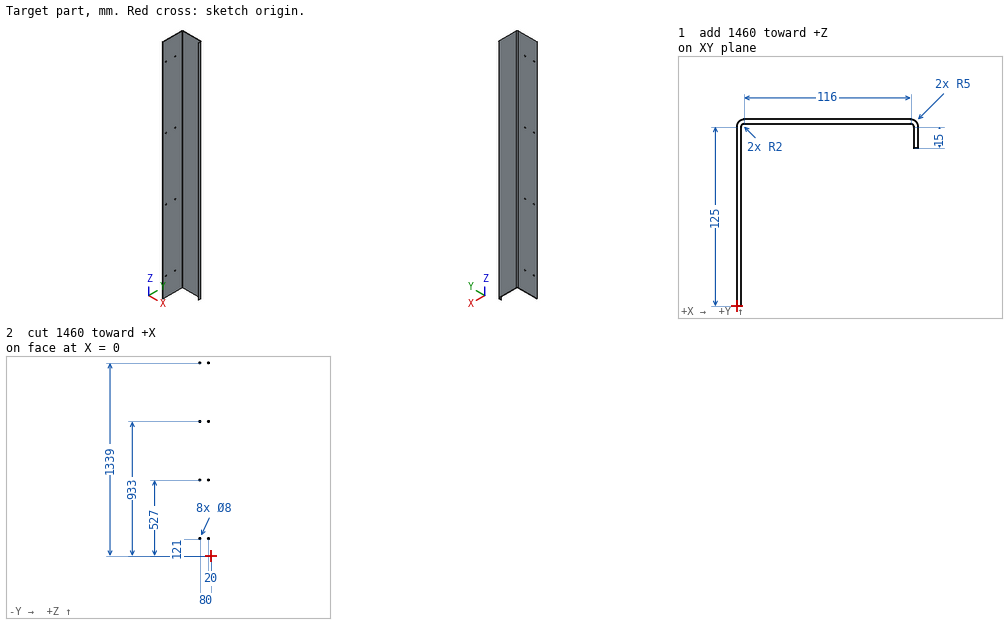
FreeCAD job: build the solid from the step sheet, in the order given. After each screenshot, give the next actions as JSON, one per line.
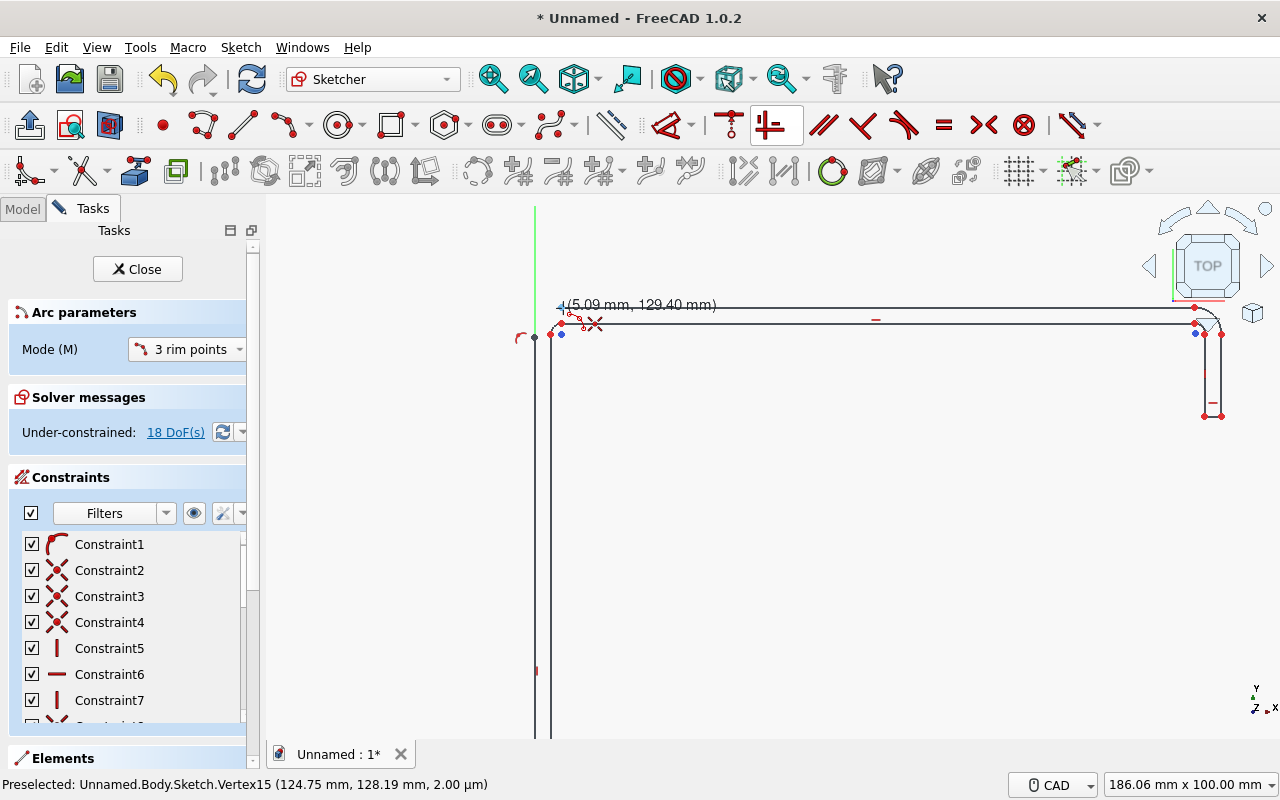
{"action": "left_click", "coordinate": [562, 308]}
{"action": "left_click", "coordinate": [535, 337]}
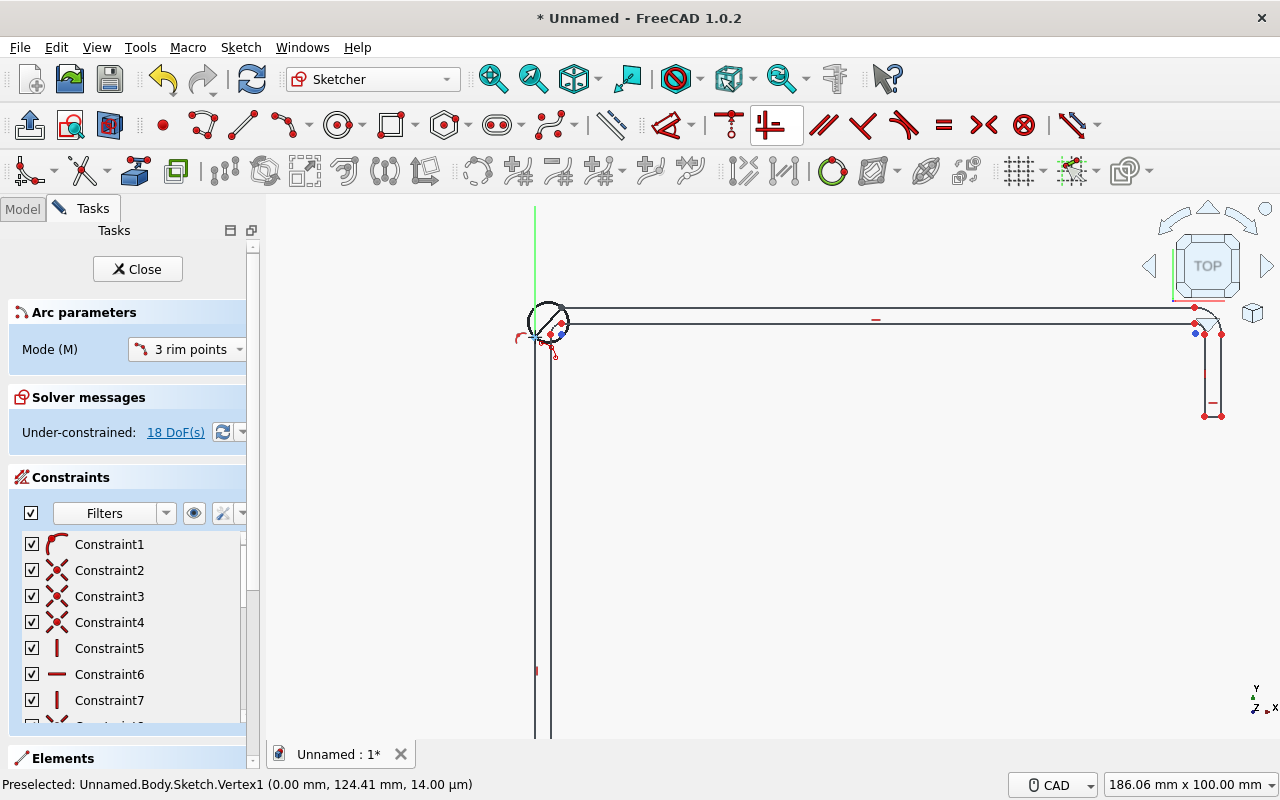
{"action": "scroll", "coordinate": [543, 315], "scroll_direction": "up", "scroll_amount": 4}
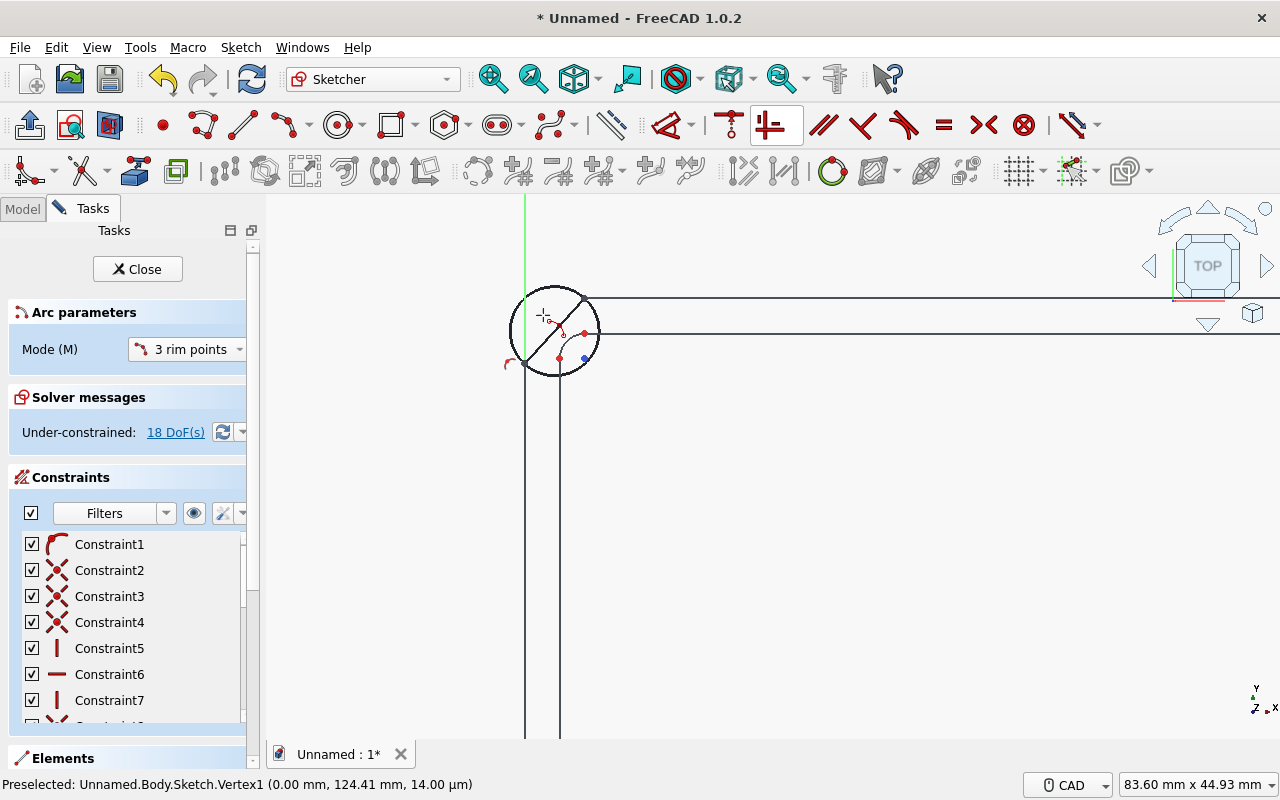
{"action": "left_click", "coordinate": [542, 314]}
{"action": "key", "text": "Escape"}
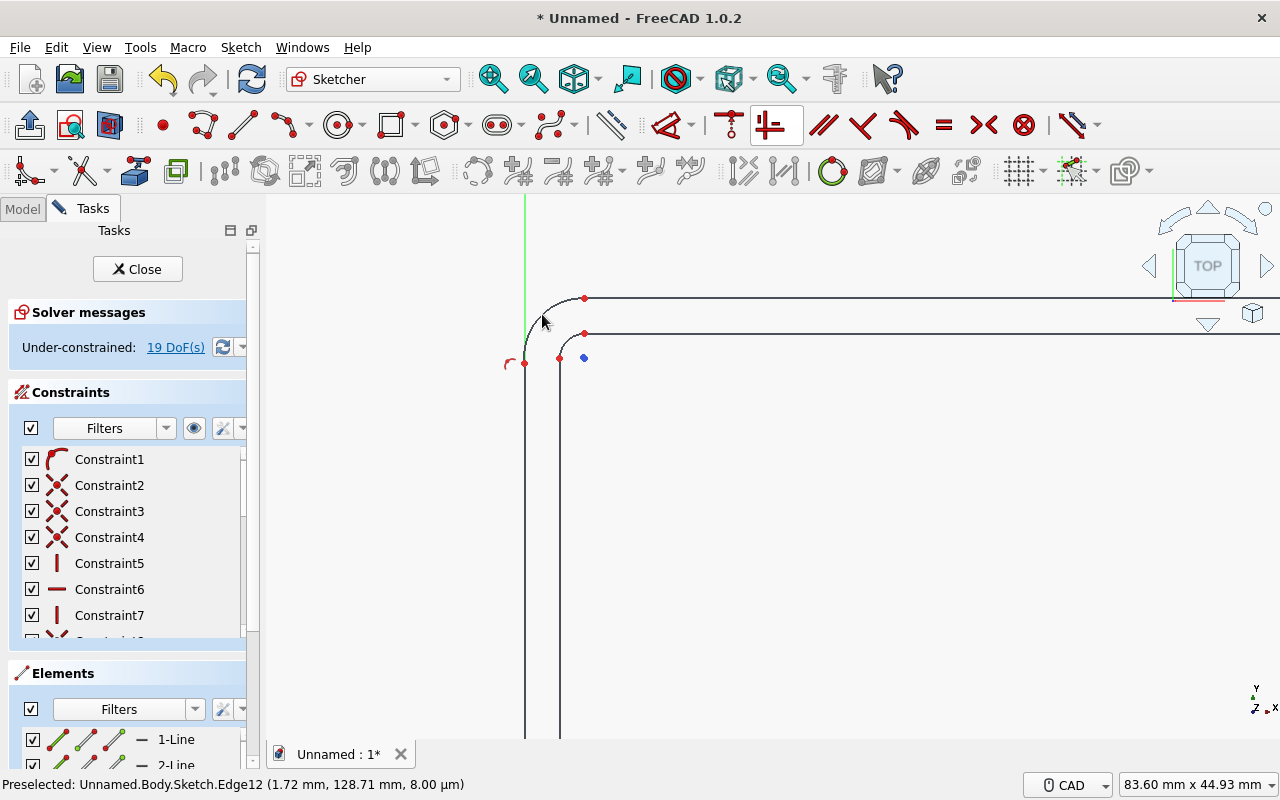
{"action": "left_click", "coordinate": [525, 666]}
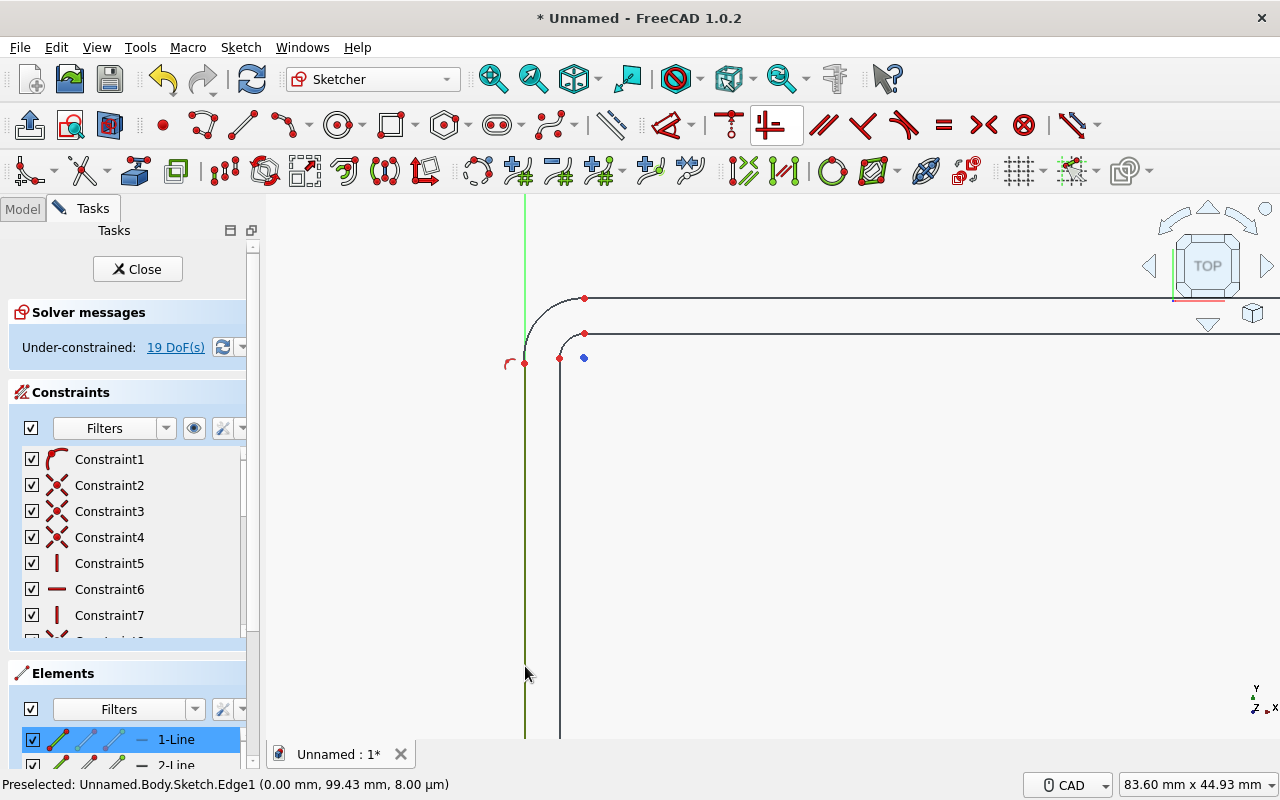
{"action": "left_click", "coordinate": [556, 305]}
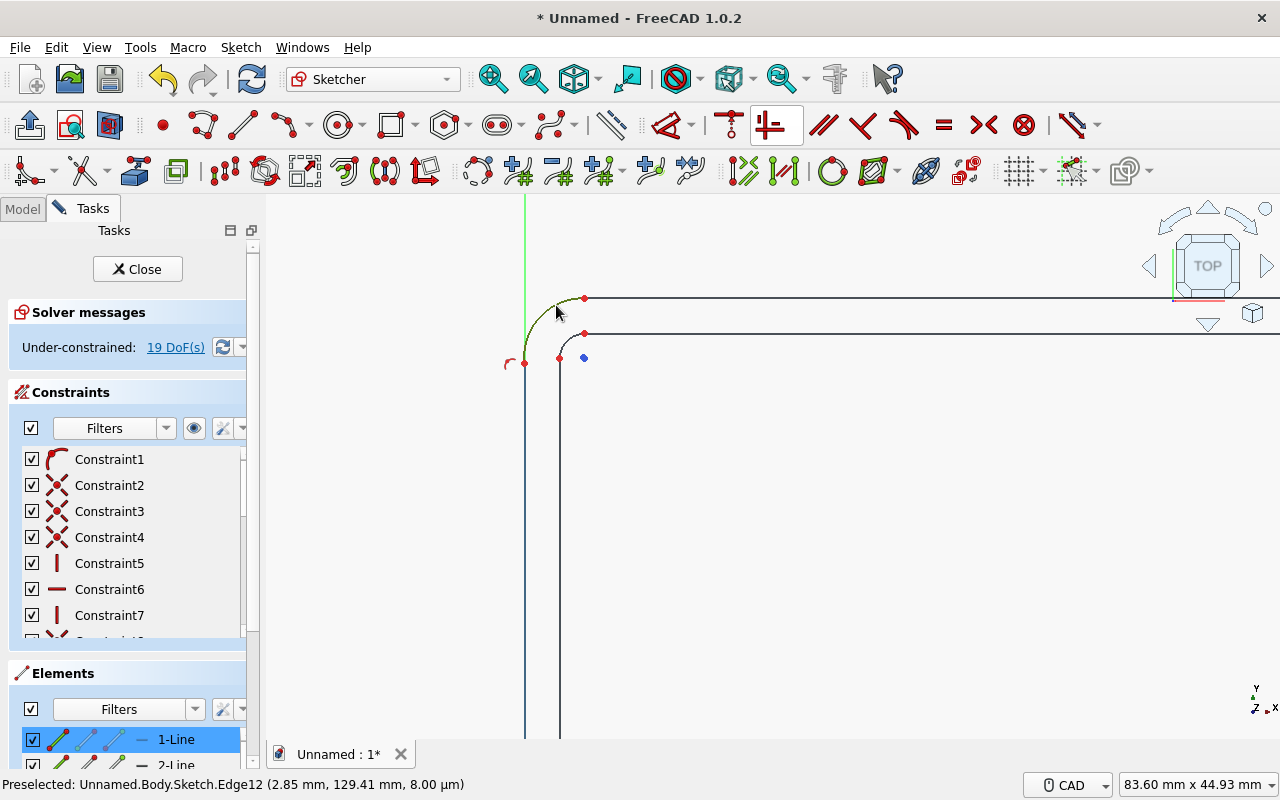
{"action": "left_click", "coordinate": [904, 126]}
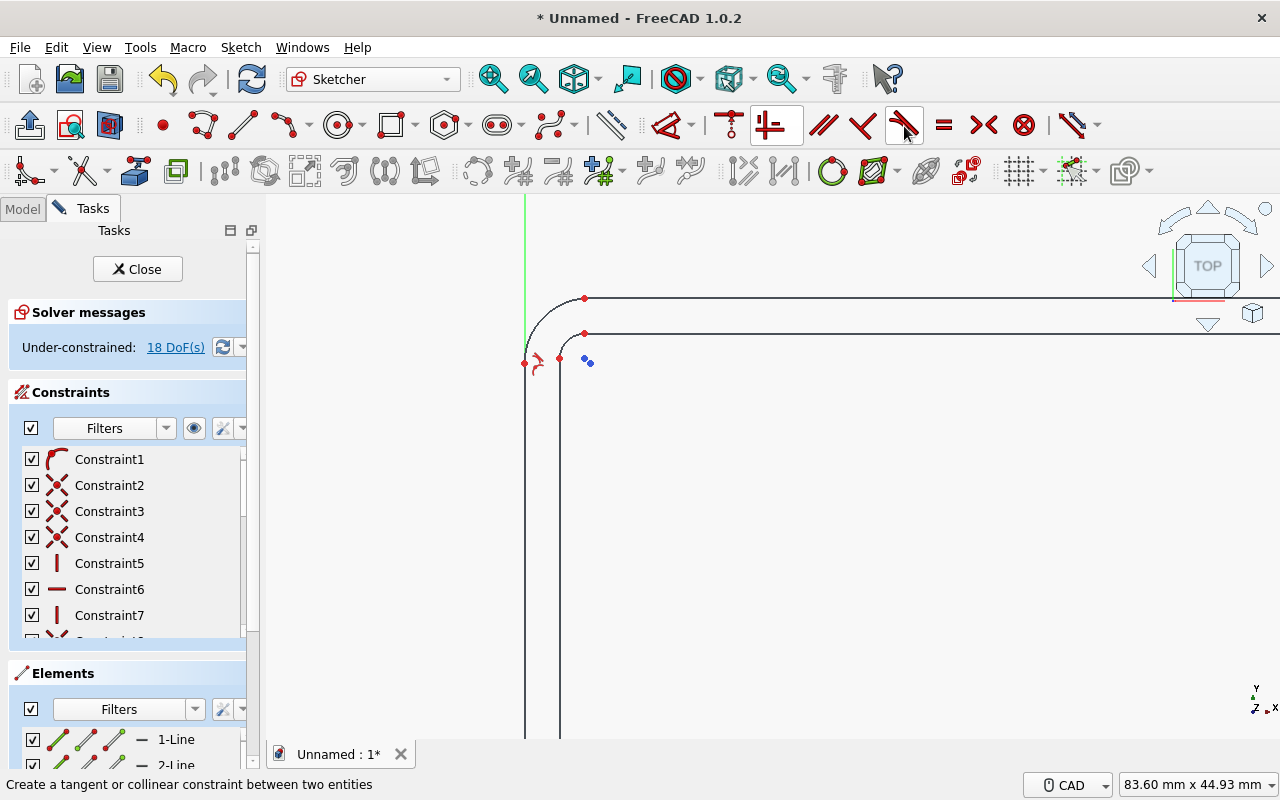
{"action": "left_click", "coordinate": [560, 658]}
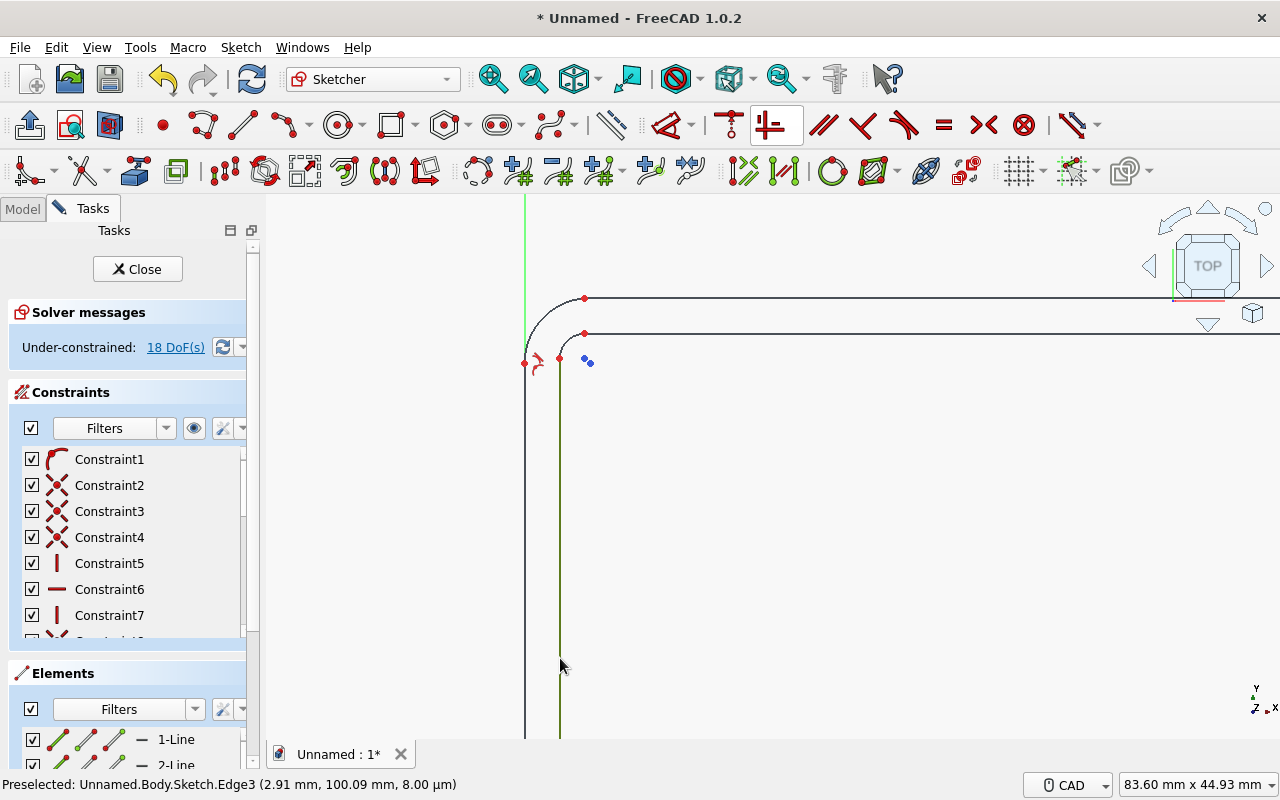
{"action": "left_click", "coordinate": [573, 337]}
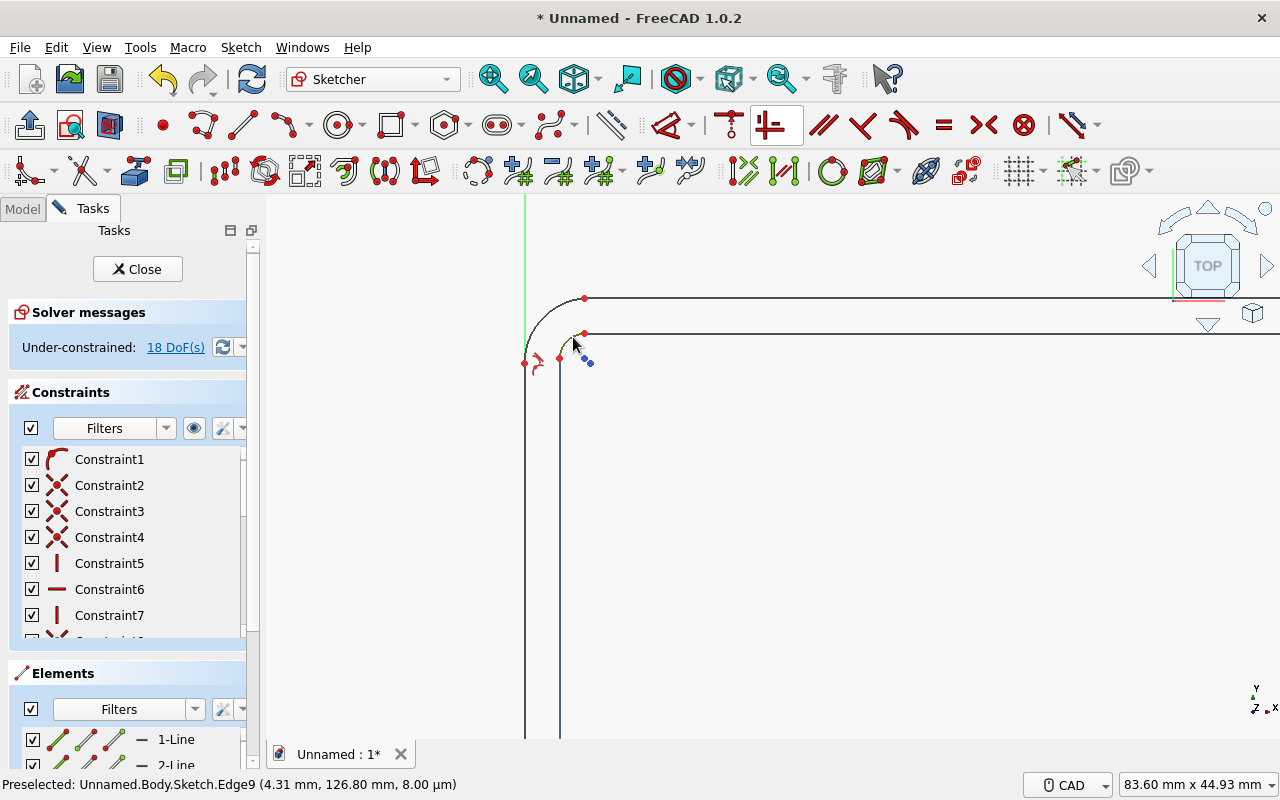
{"action": "left_click", "coordinate": [904, 126]}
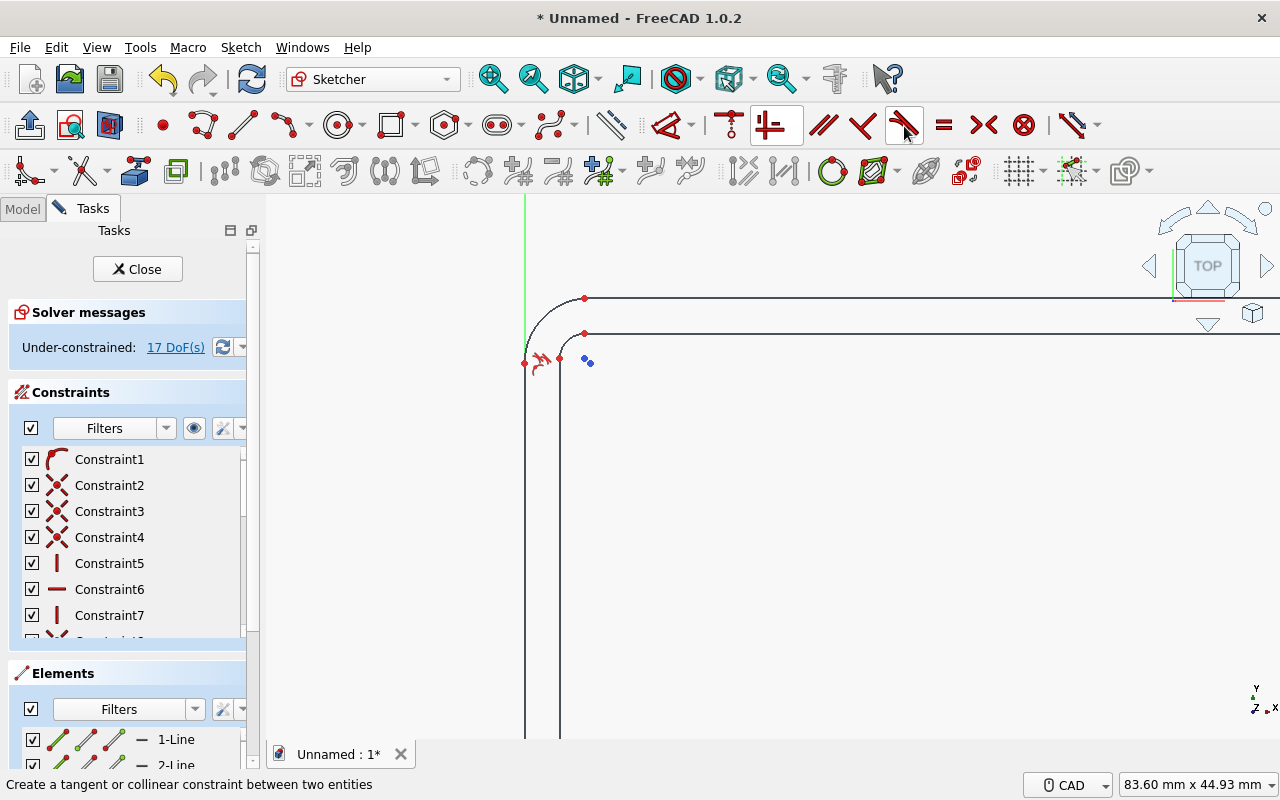
{"action": "left_click", "coordinate": [1007, 334]}